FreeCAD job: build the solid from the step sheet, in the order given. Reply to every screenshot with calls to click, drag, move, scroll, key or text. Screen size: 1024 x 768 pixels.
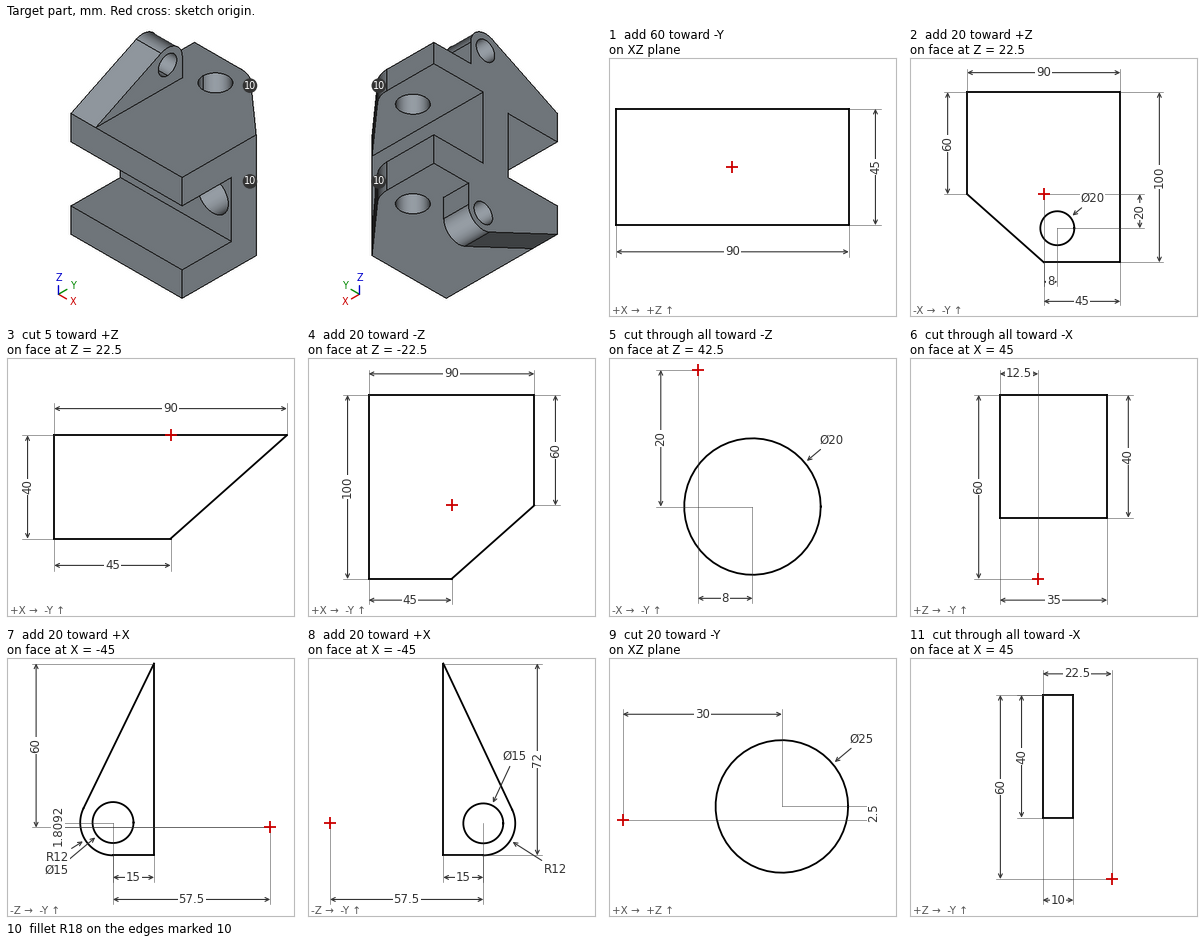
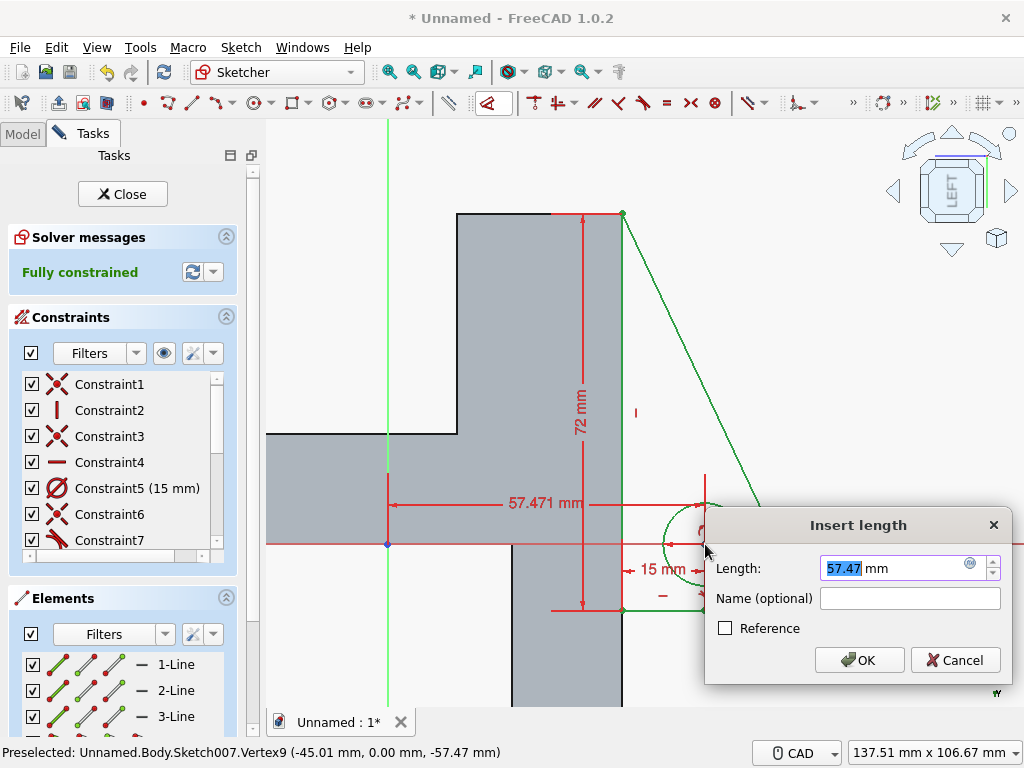
text(57.5)
key(Return)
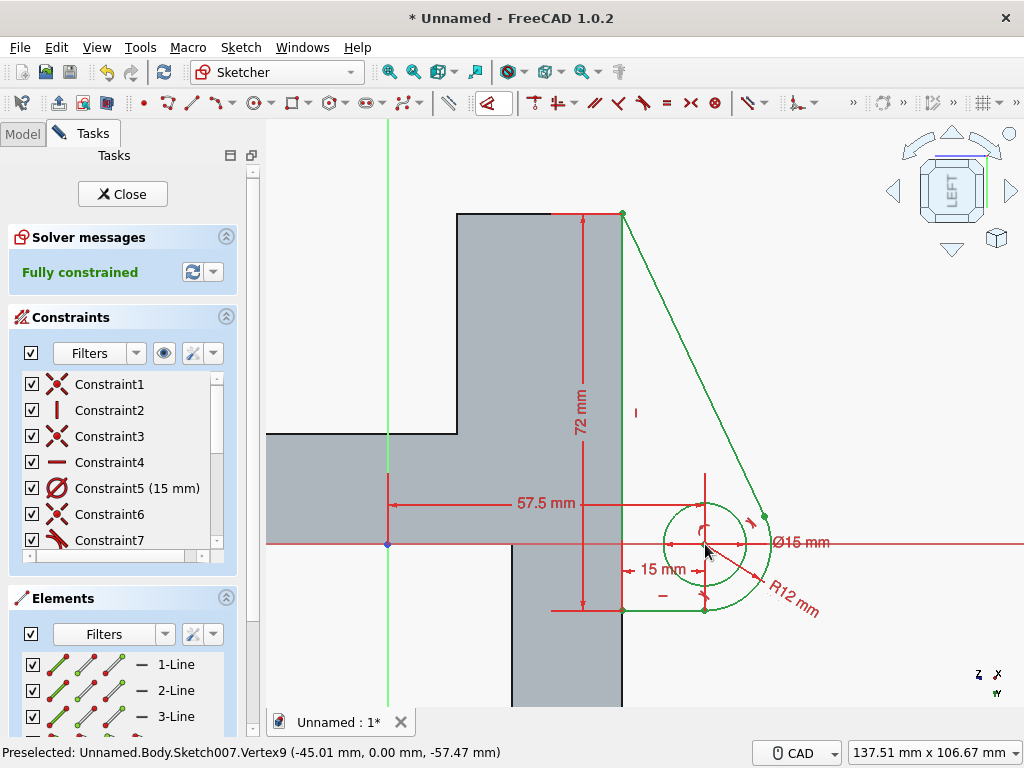
click(123, 194)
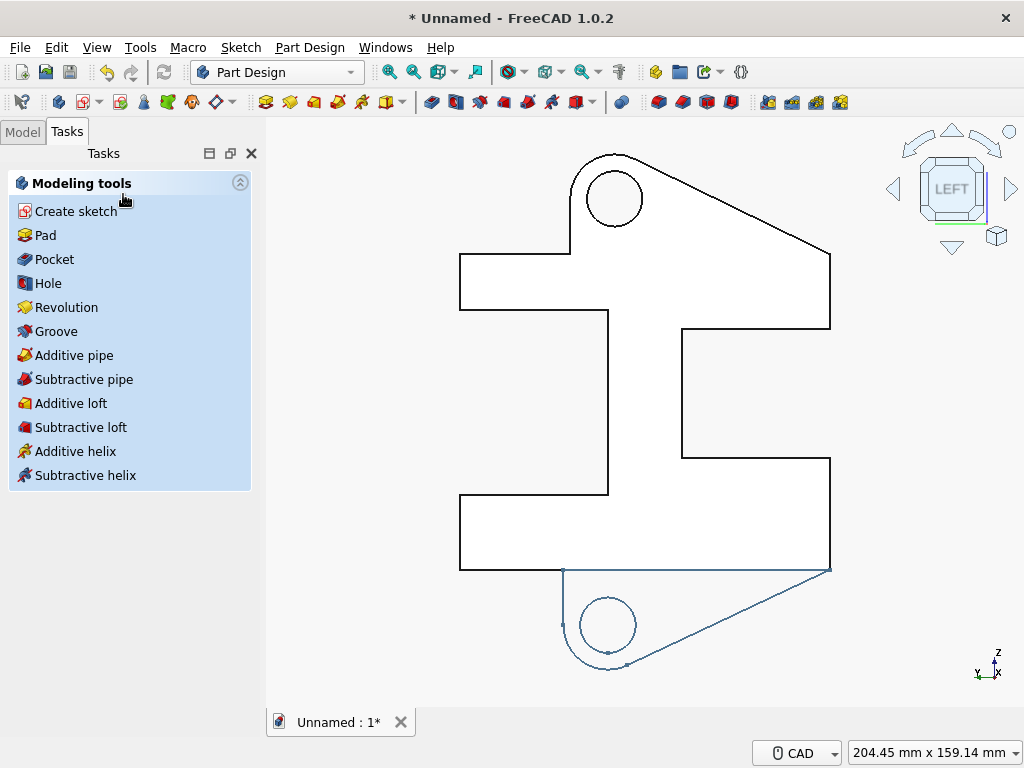
click(266, 102)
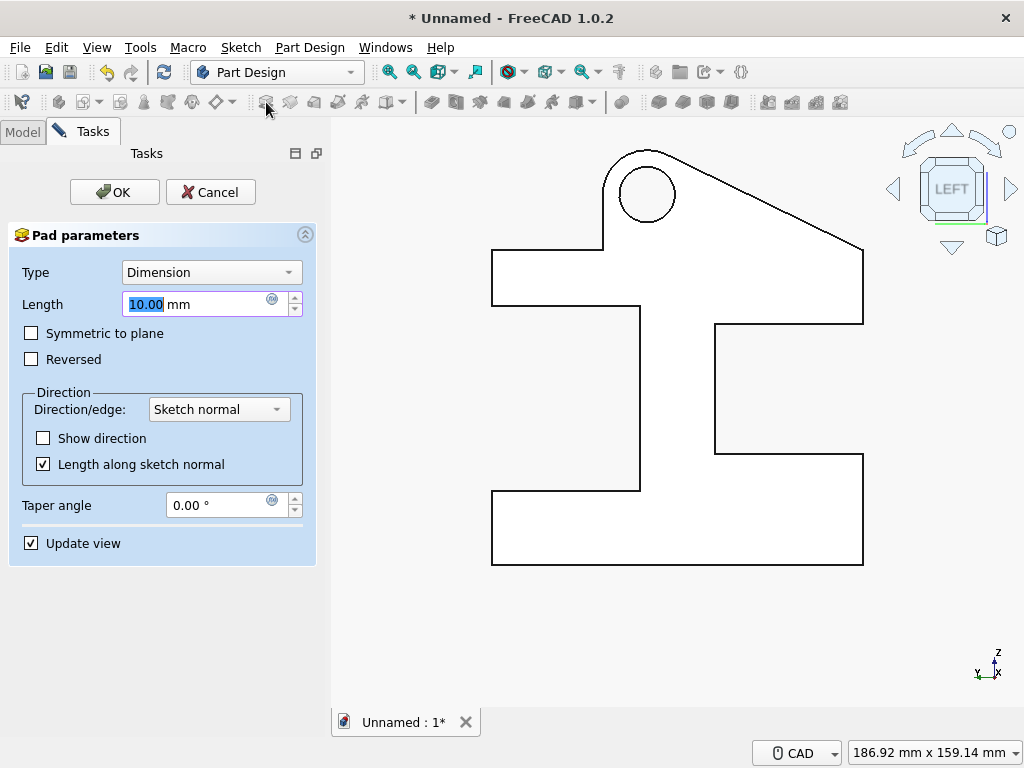
text(20)
key(Tab)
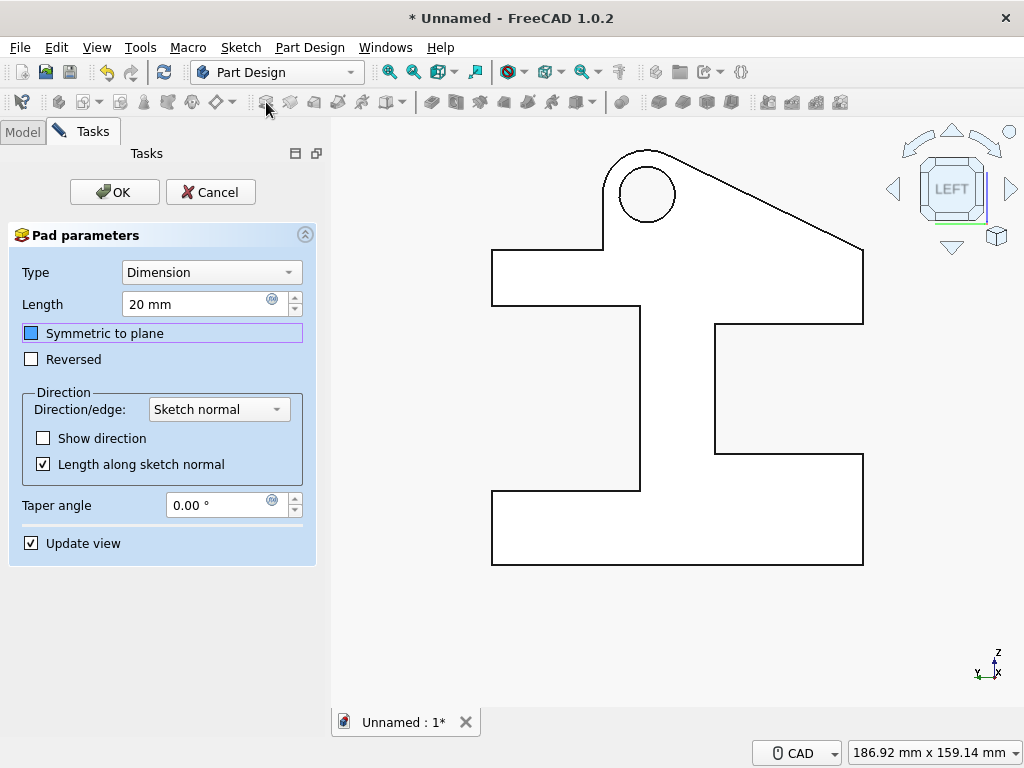
click(30, 359)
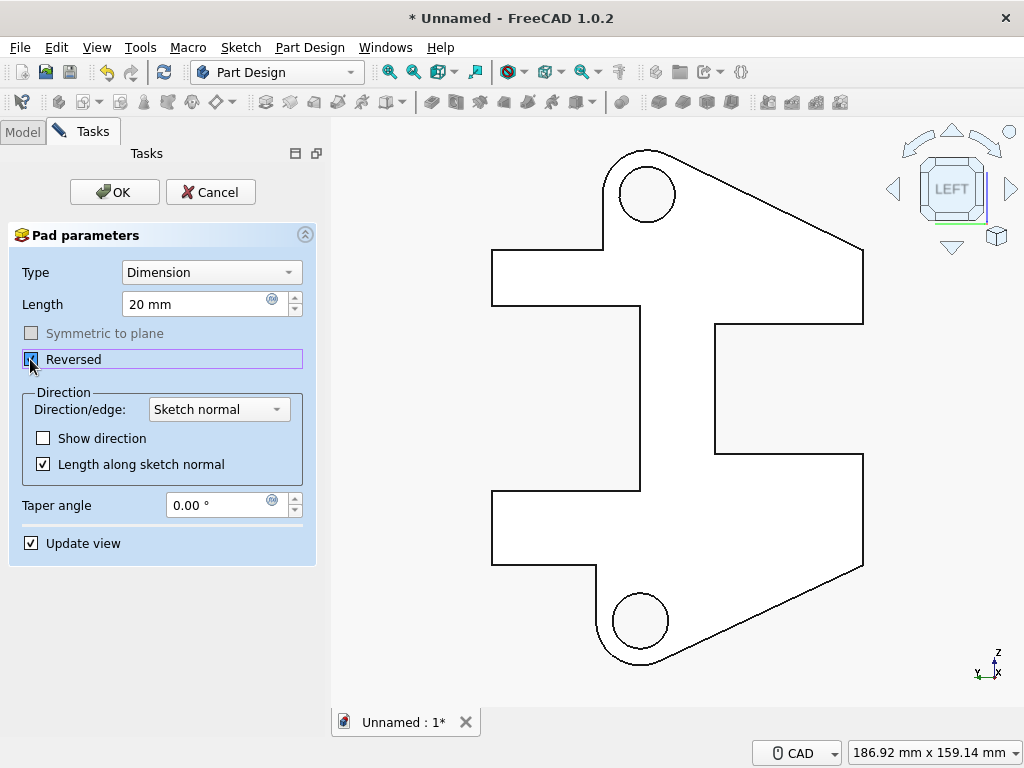
click(115, 192)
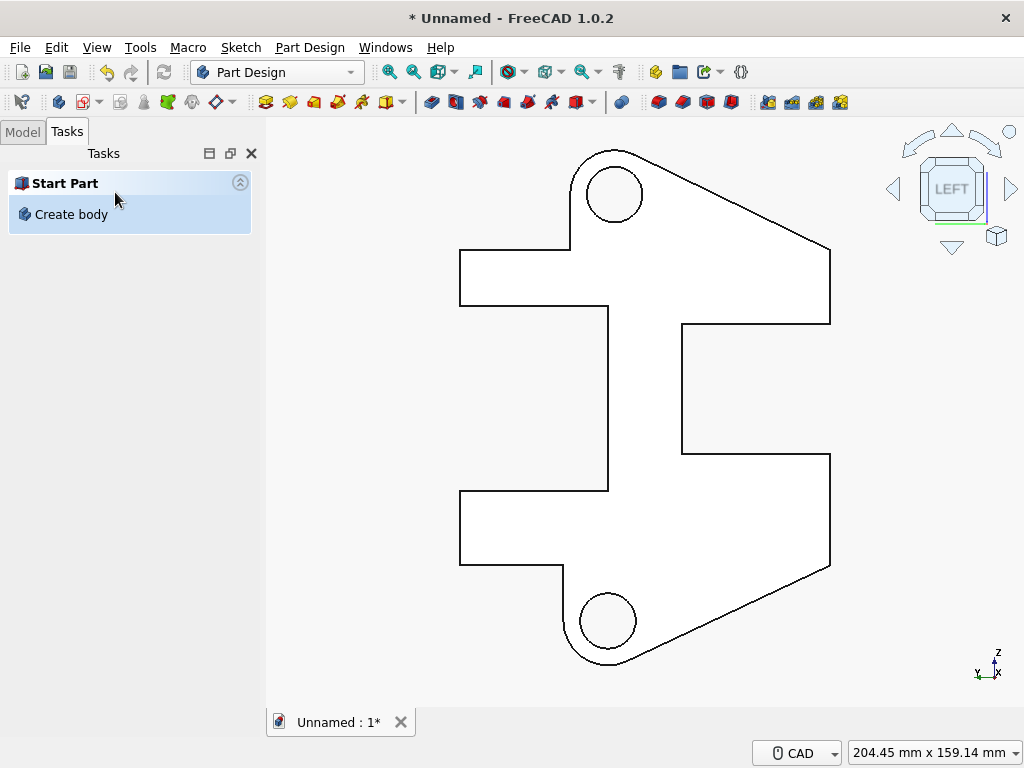
click(84, 102)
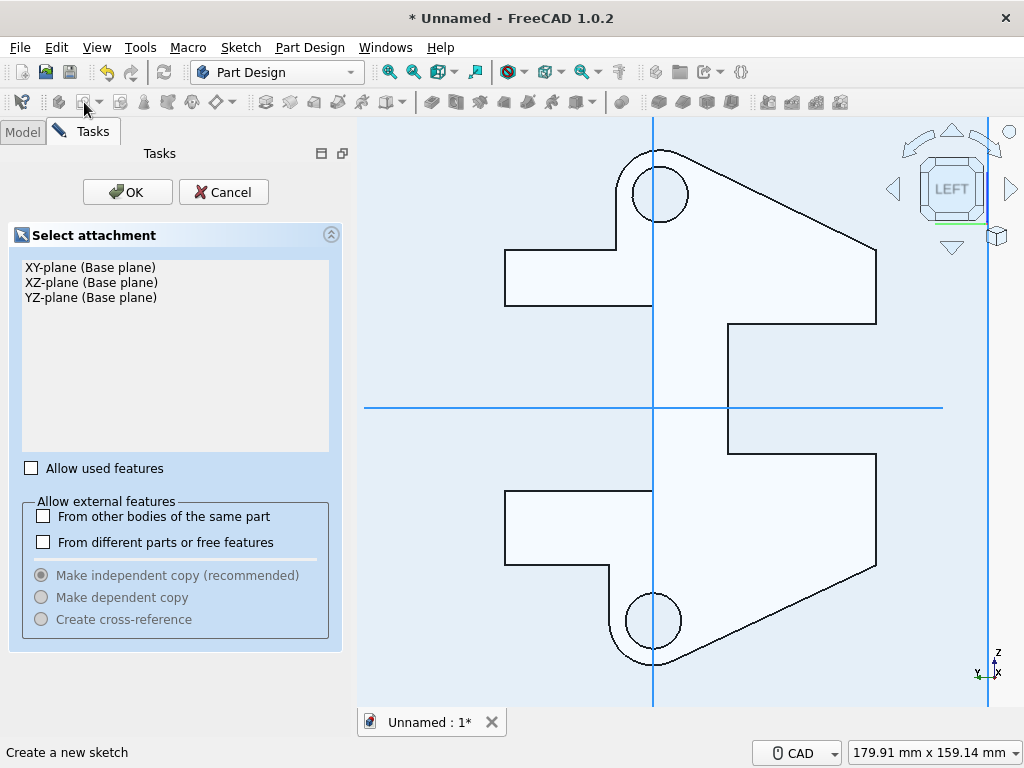
click(82, 282)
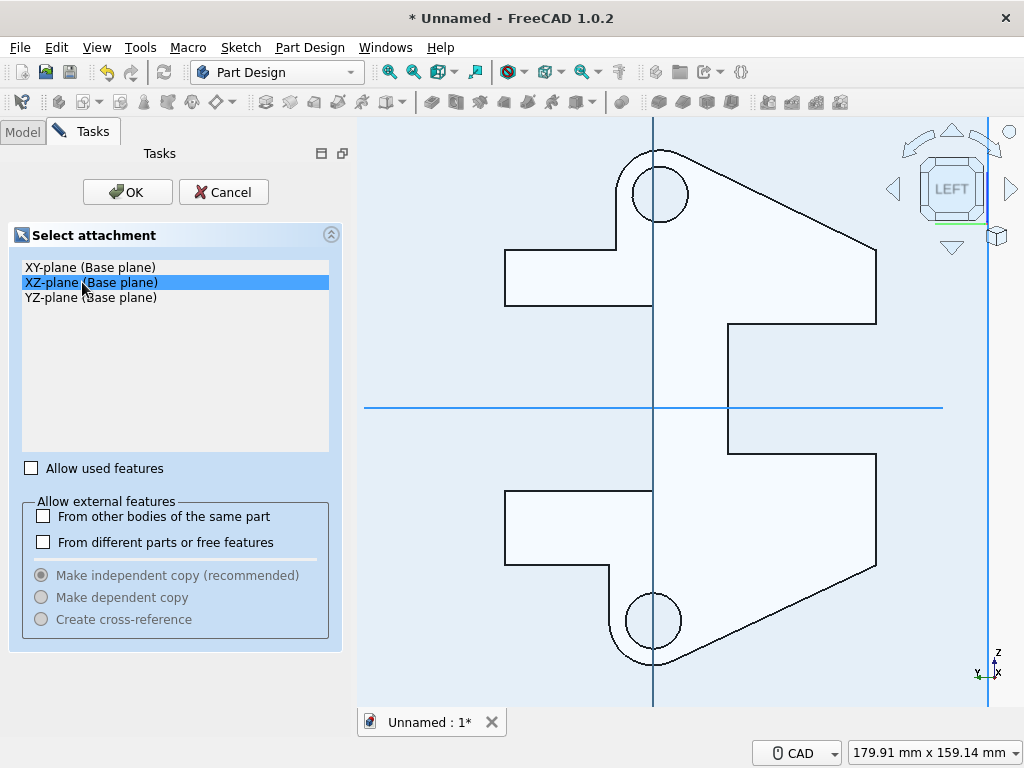
click(128, 192)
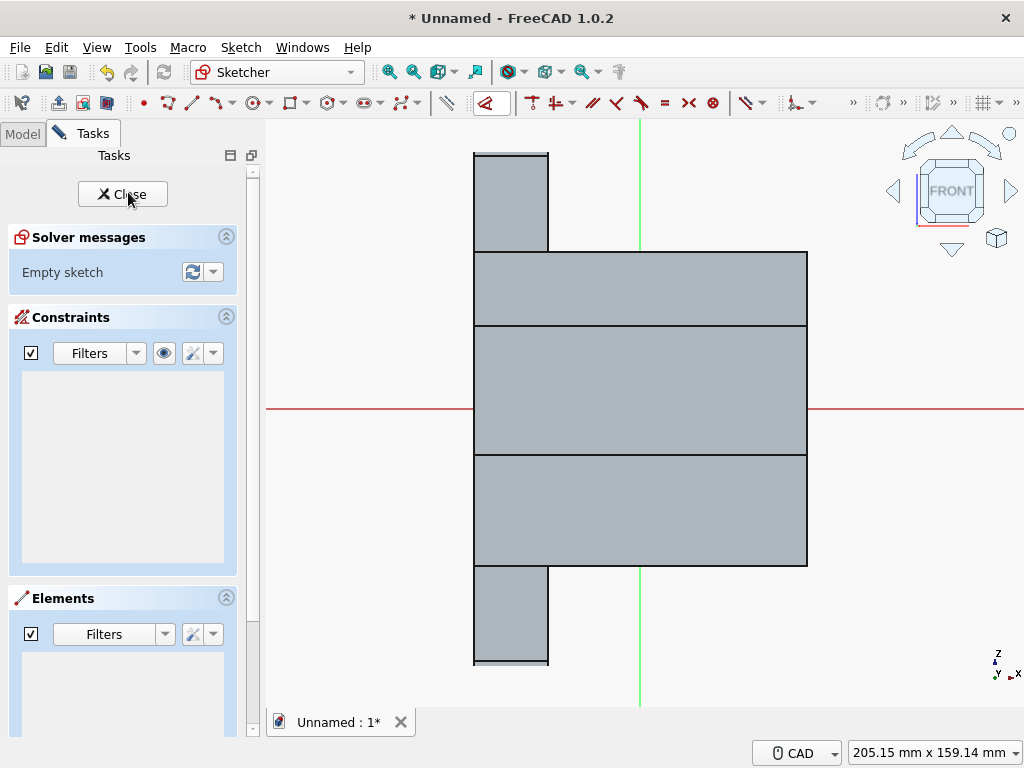
key(q)
key(s)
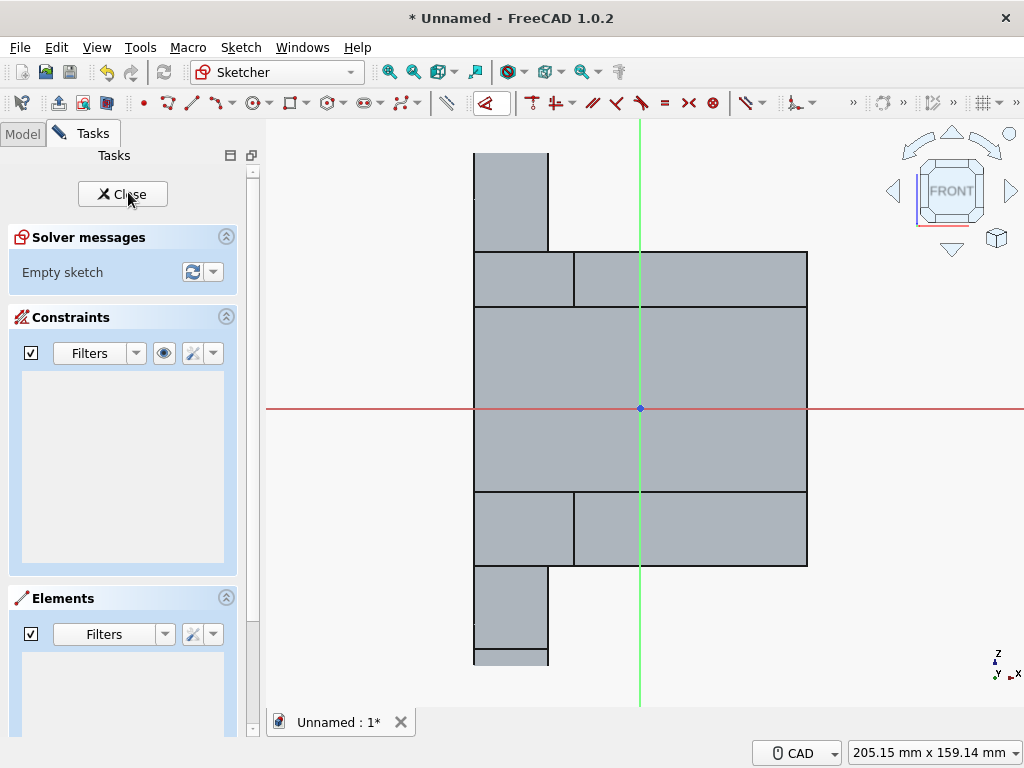
scroll(802, 392, up, 5)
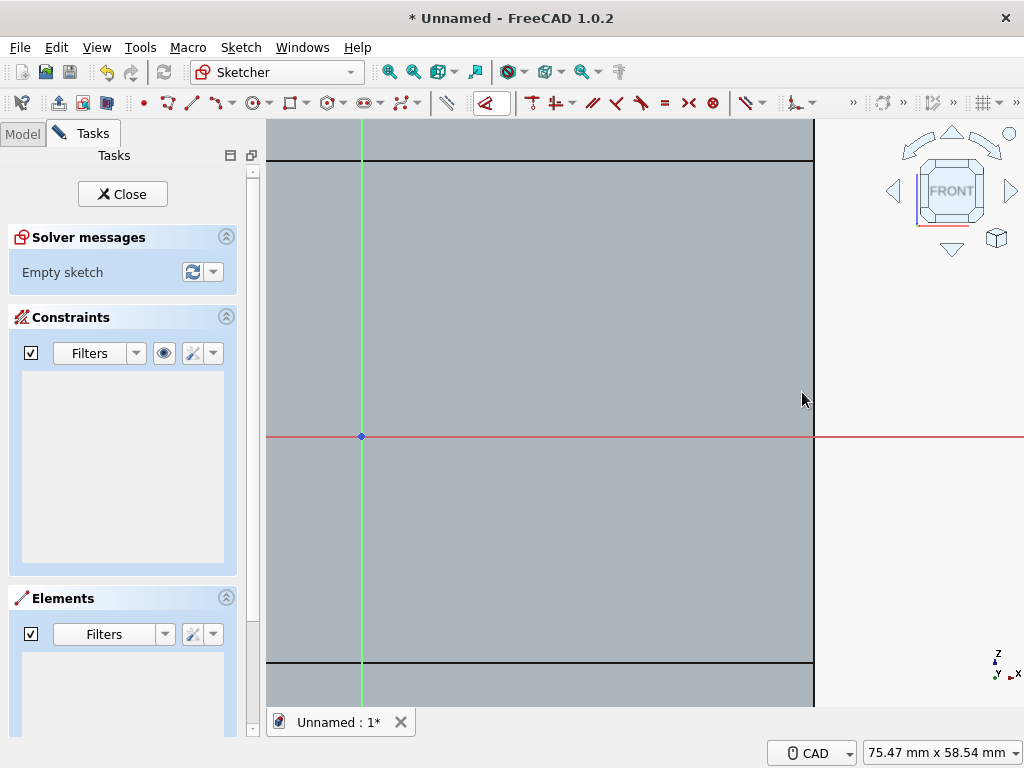
key(g)
key(c)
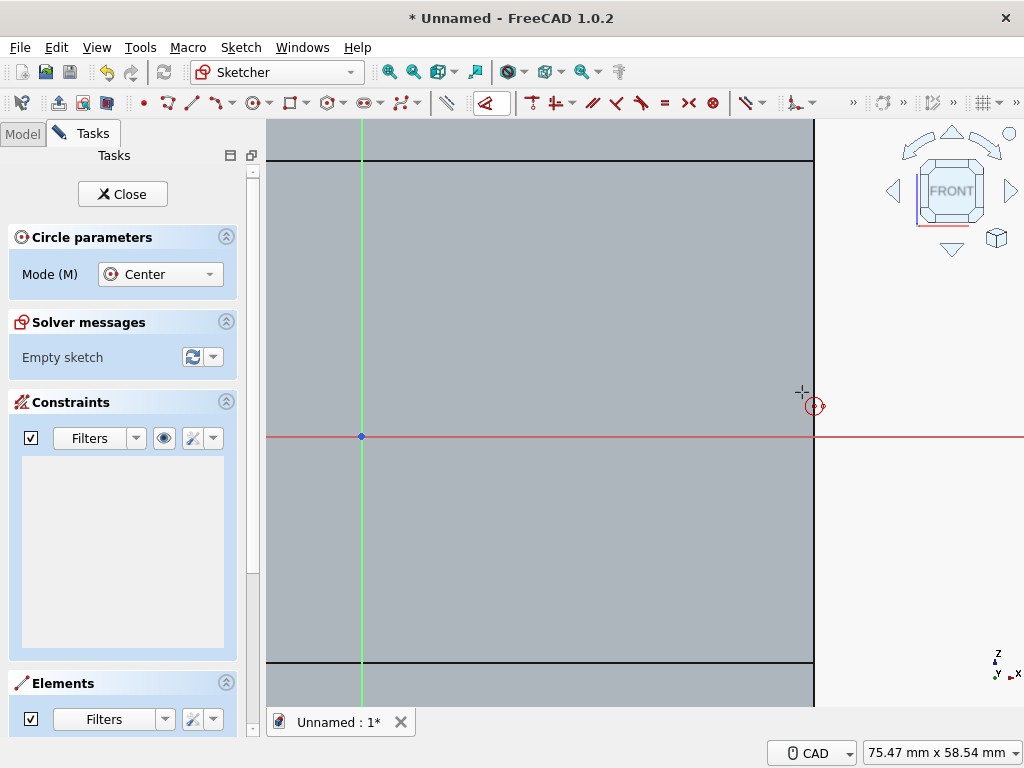
click(663, 412)
move(752, 323)